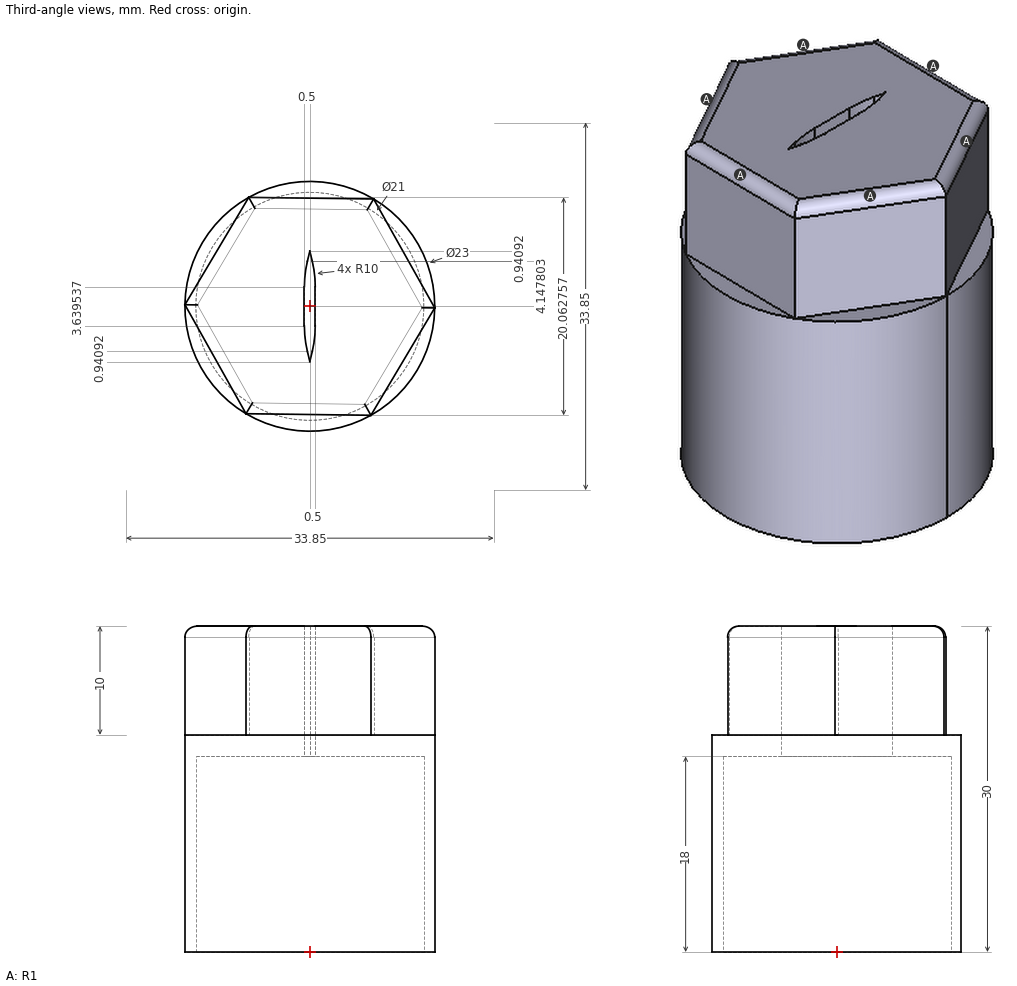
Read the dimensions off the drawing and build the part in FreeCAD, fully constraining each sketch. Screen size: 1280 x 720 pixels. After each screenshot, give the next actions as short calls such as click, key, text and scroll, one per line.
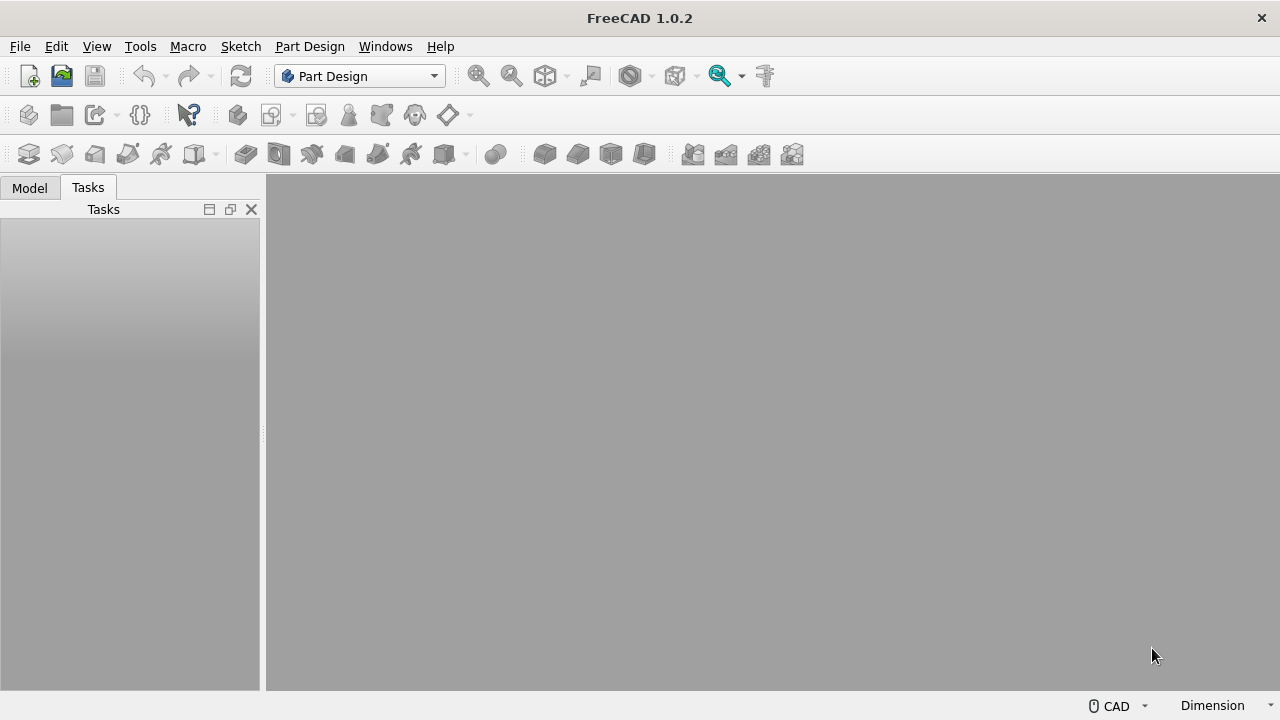
click(29, 76)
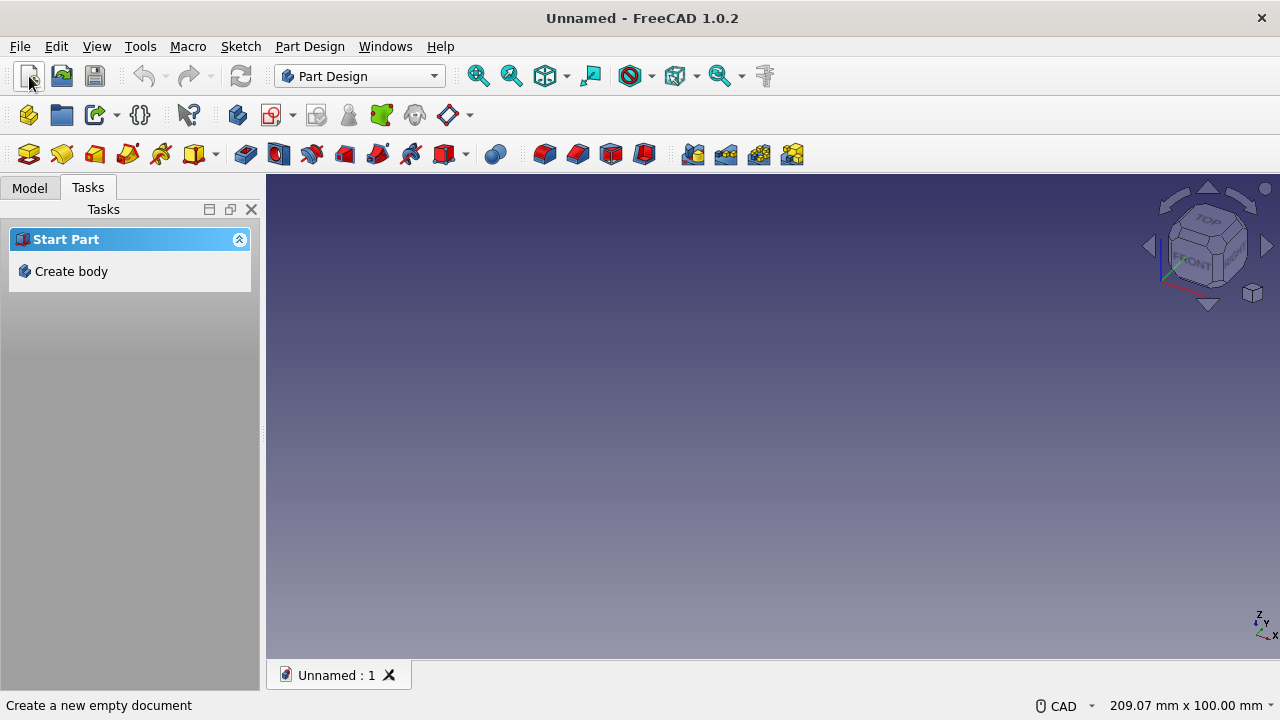
click(270, 116)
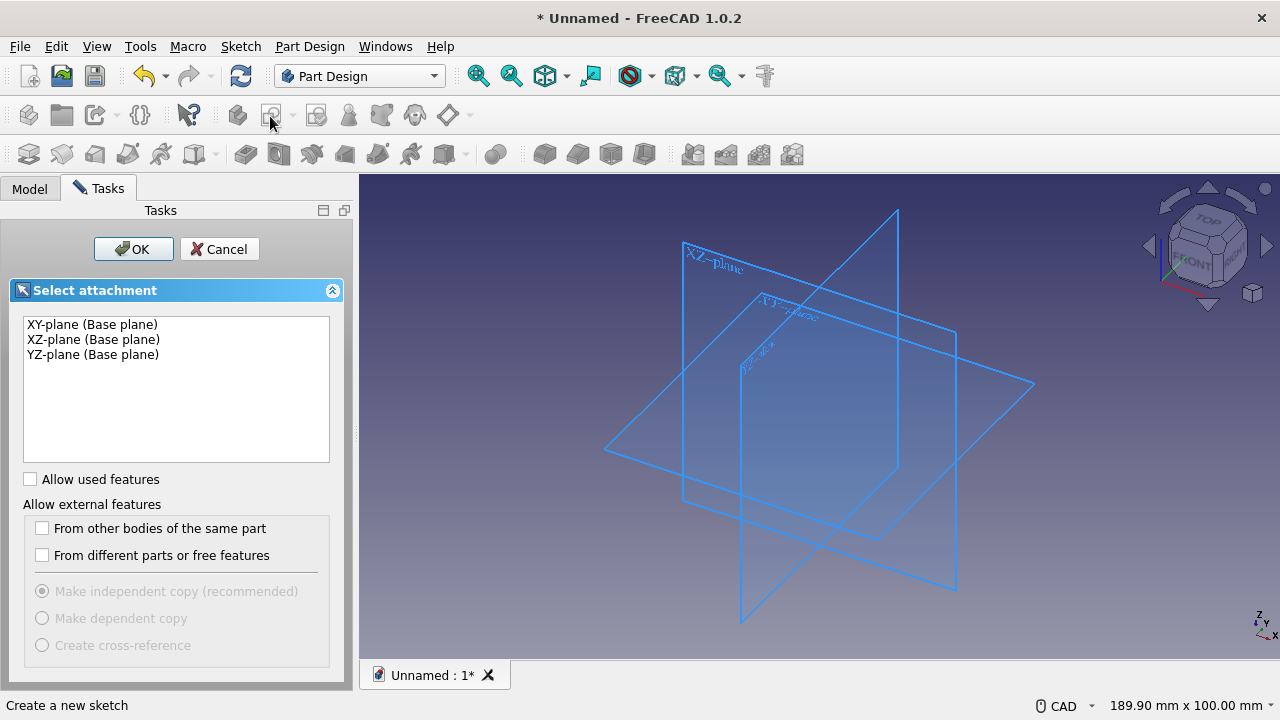
click(84, 324)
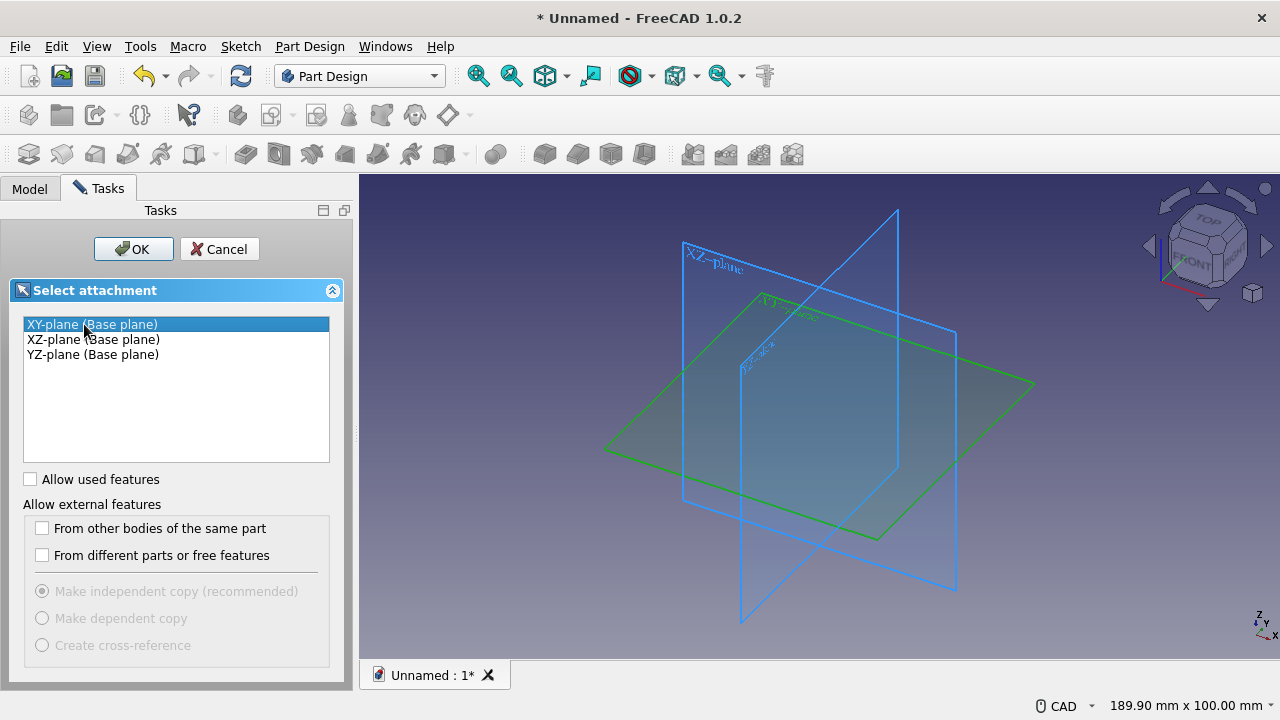
click(134, 249)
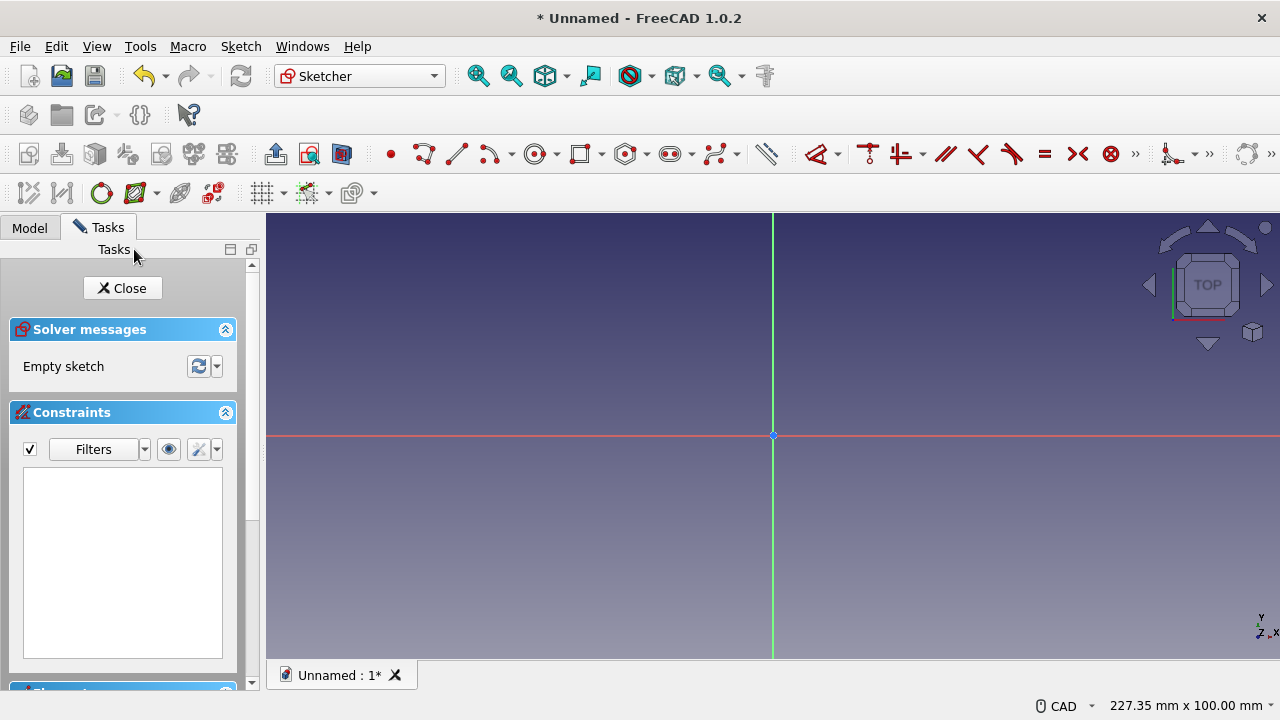
scroll(813, 436, up, 5)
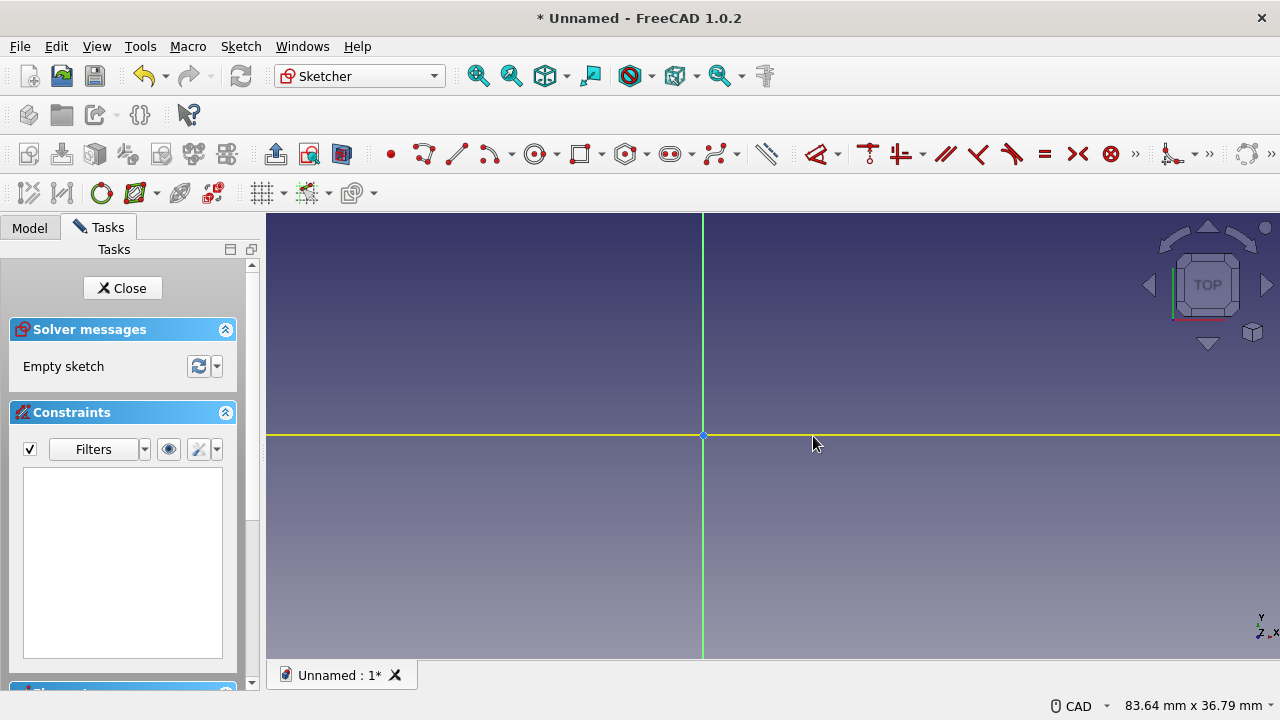
click(534, 154)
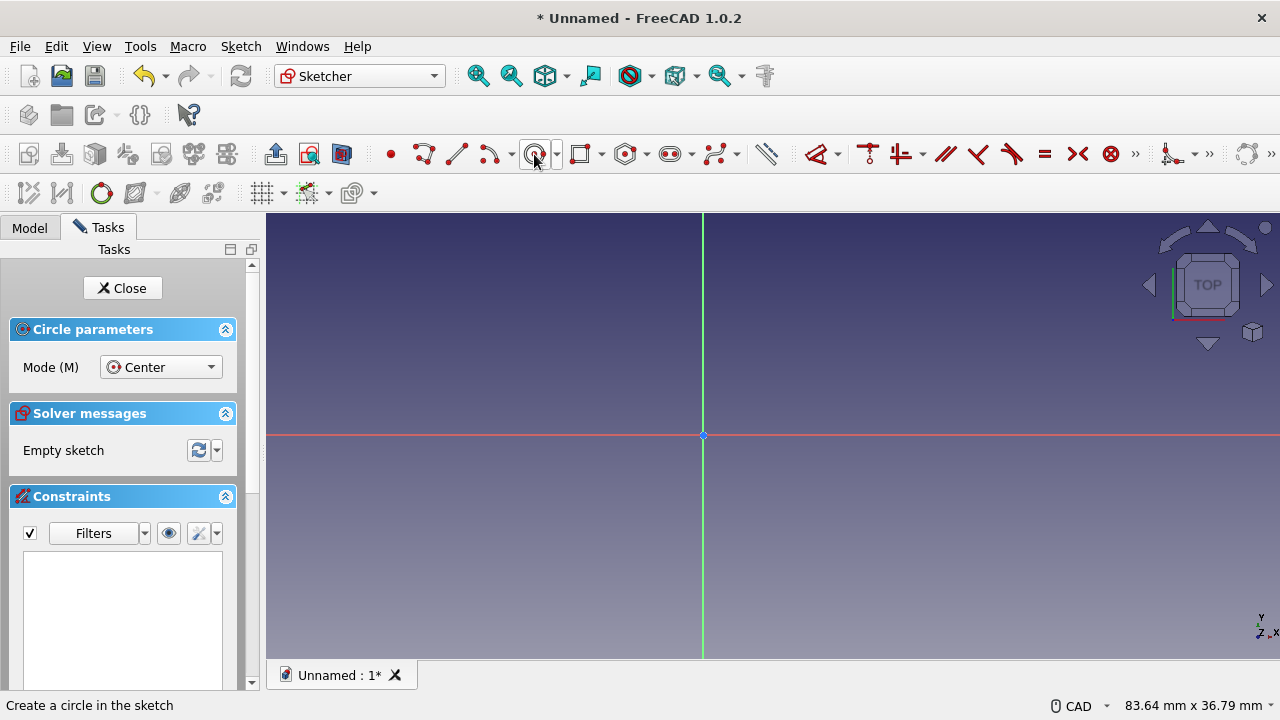
click(703, 435)
click(802, 337)
key(Escape)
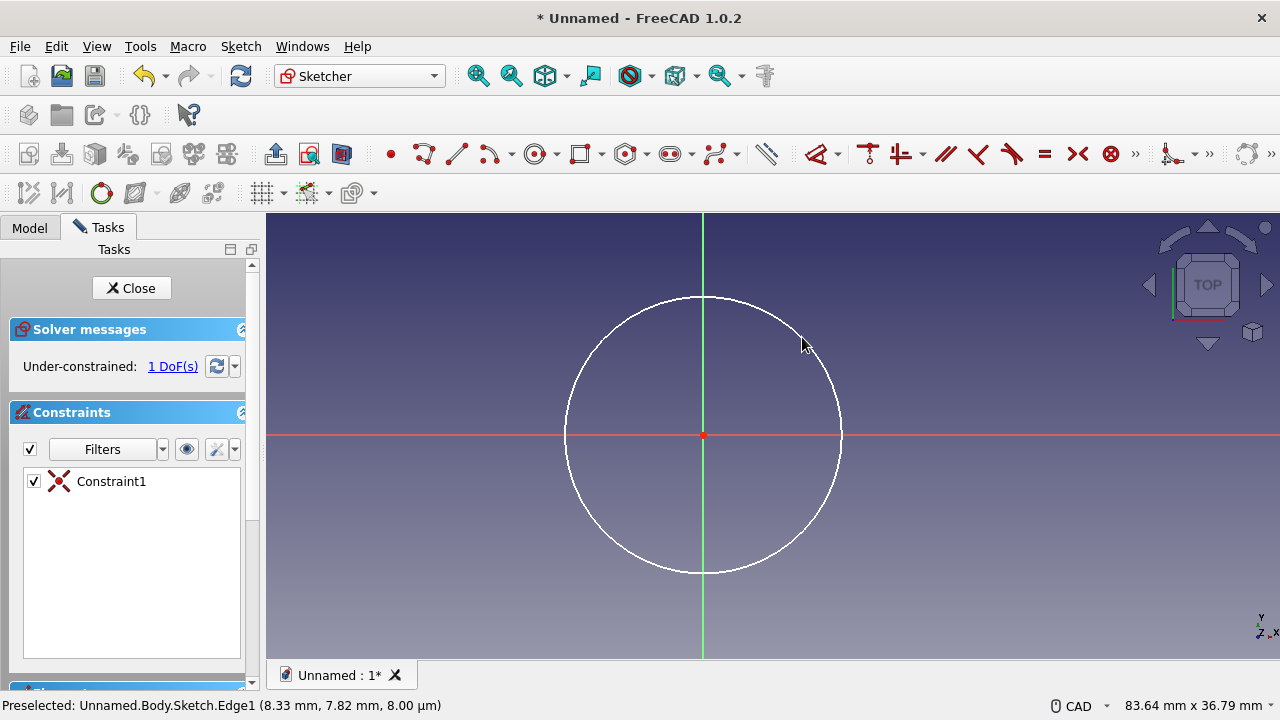
click(801, 337)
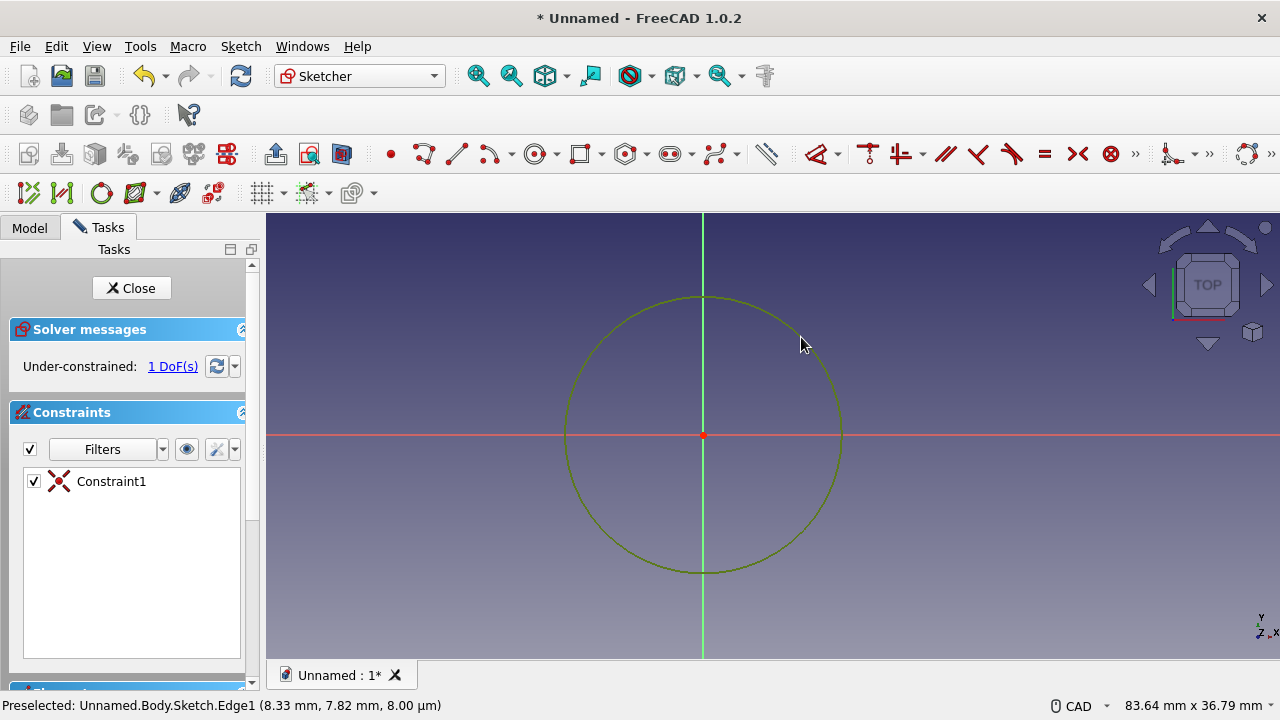
key(k)
key(o)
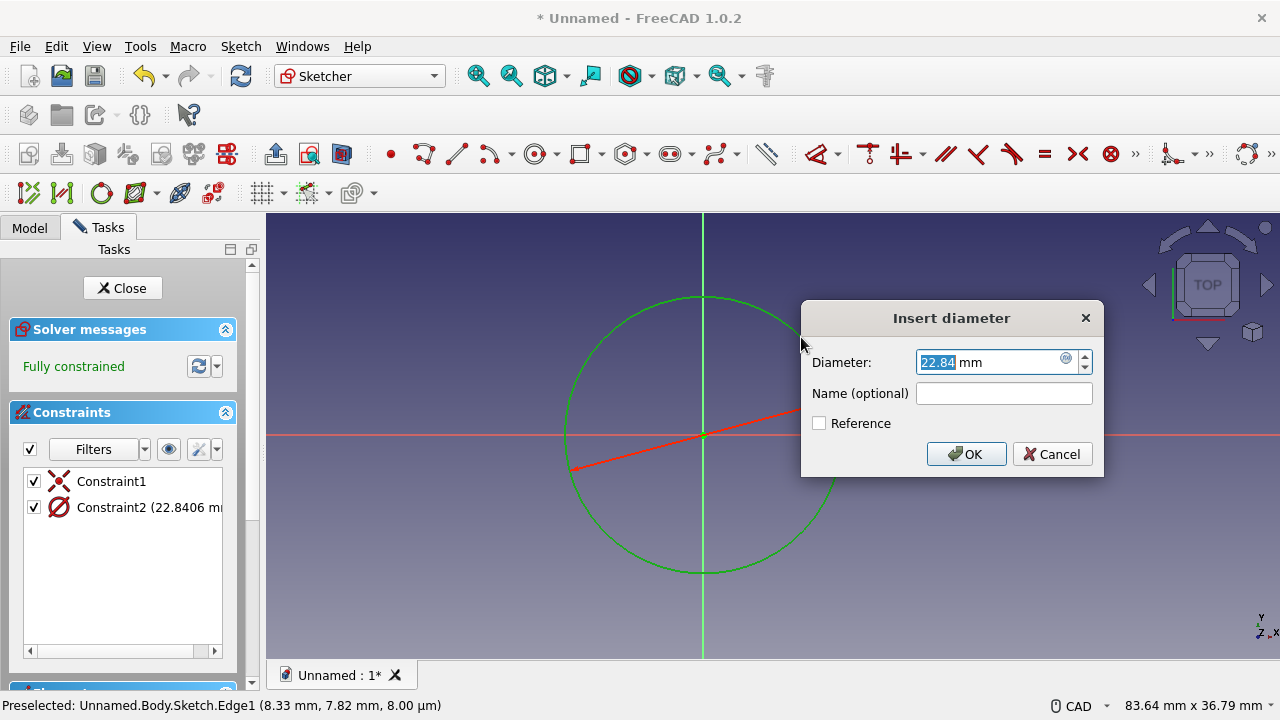
text(23)
key(Return)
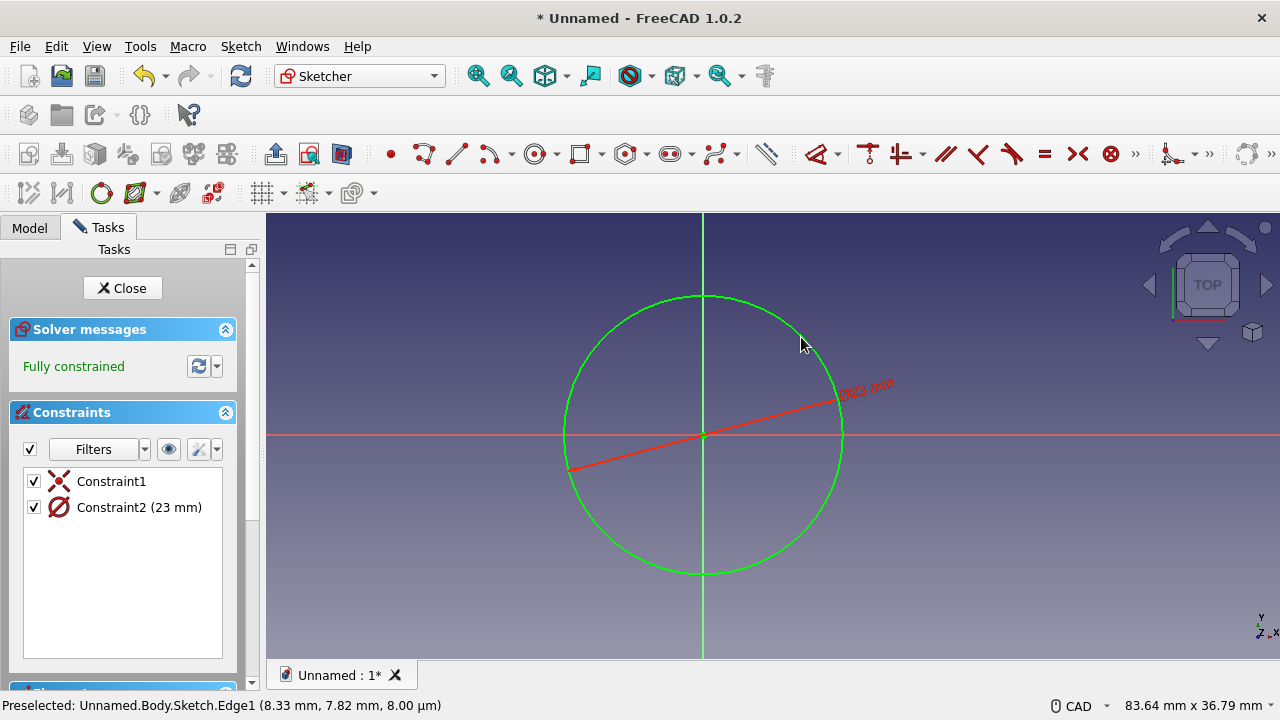
click(123, 288)